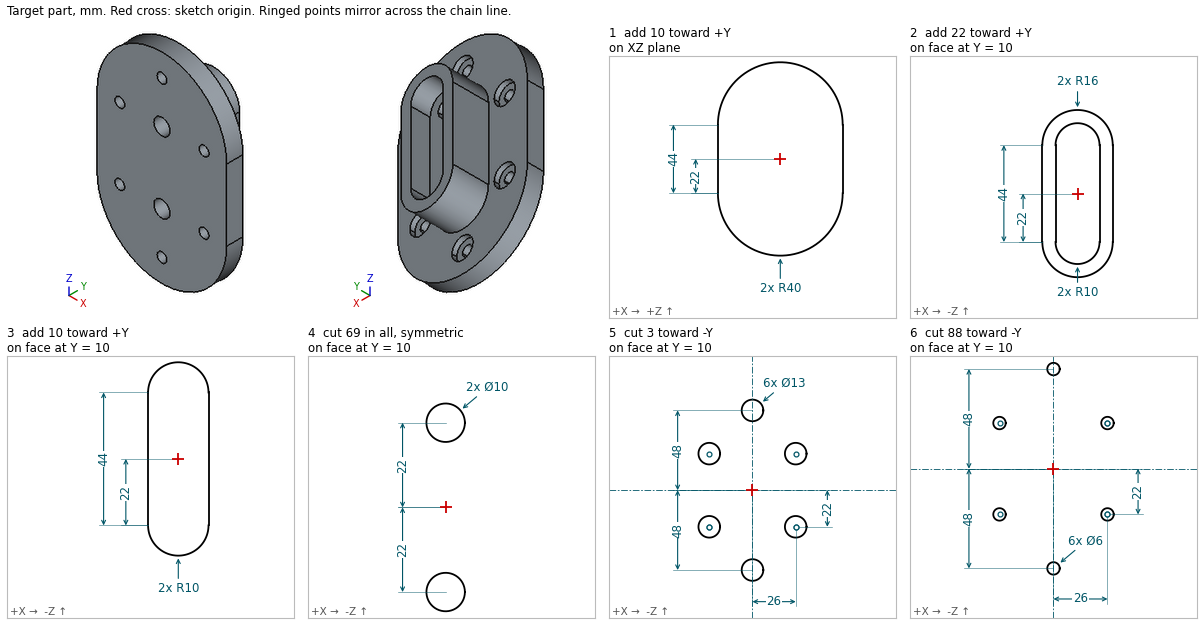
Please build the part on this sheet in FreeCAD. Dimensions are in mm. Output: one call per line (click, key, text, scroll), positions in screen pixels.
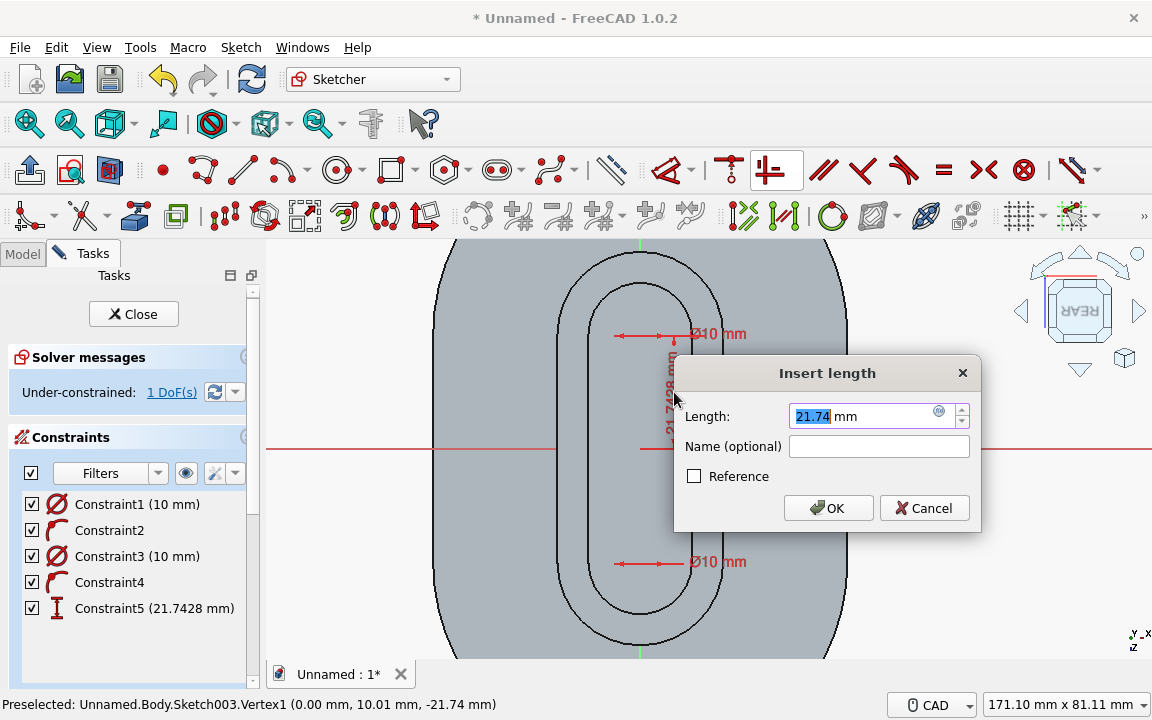
text(22)
key(Return)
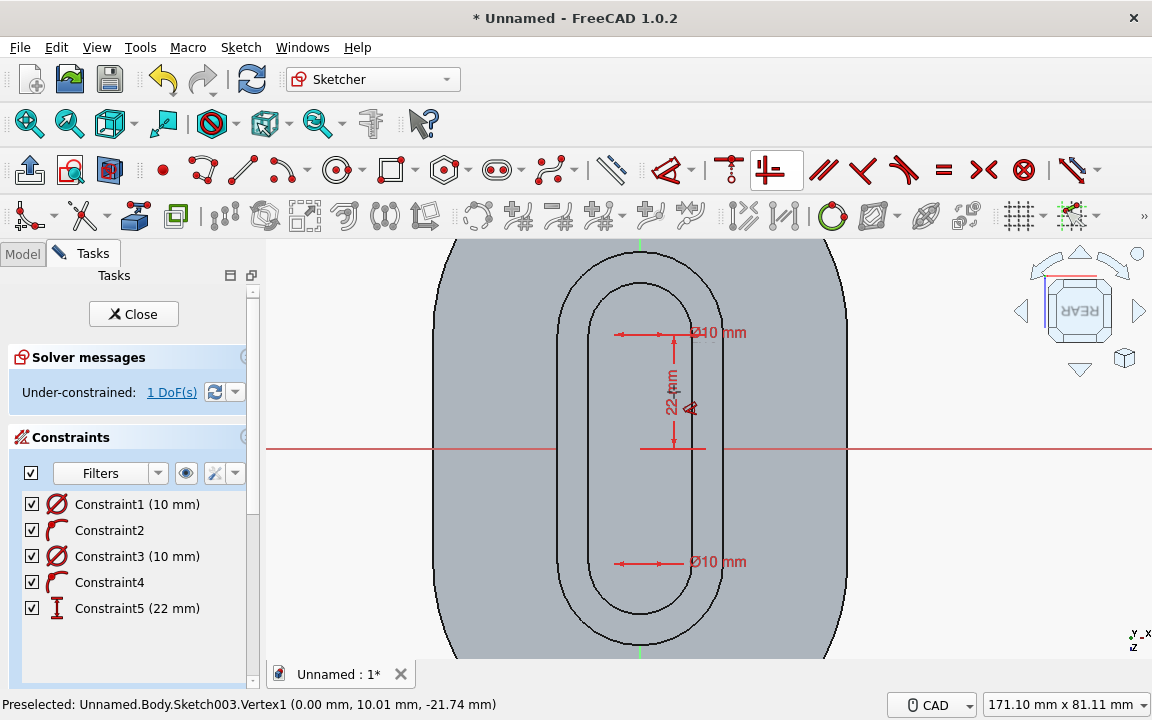
click(640, 564)
click(674, 506)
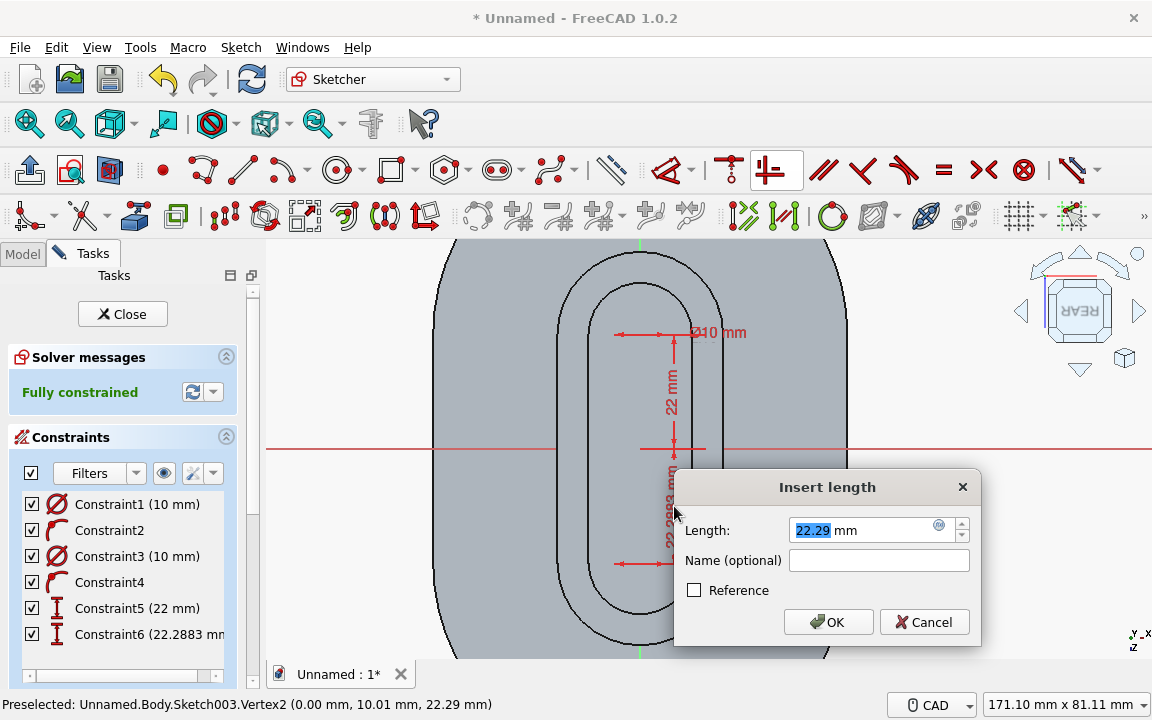
text(22)
key(Return)
key(Escape)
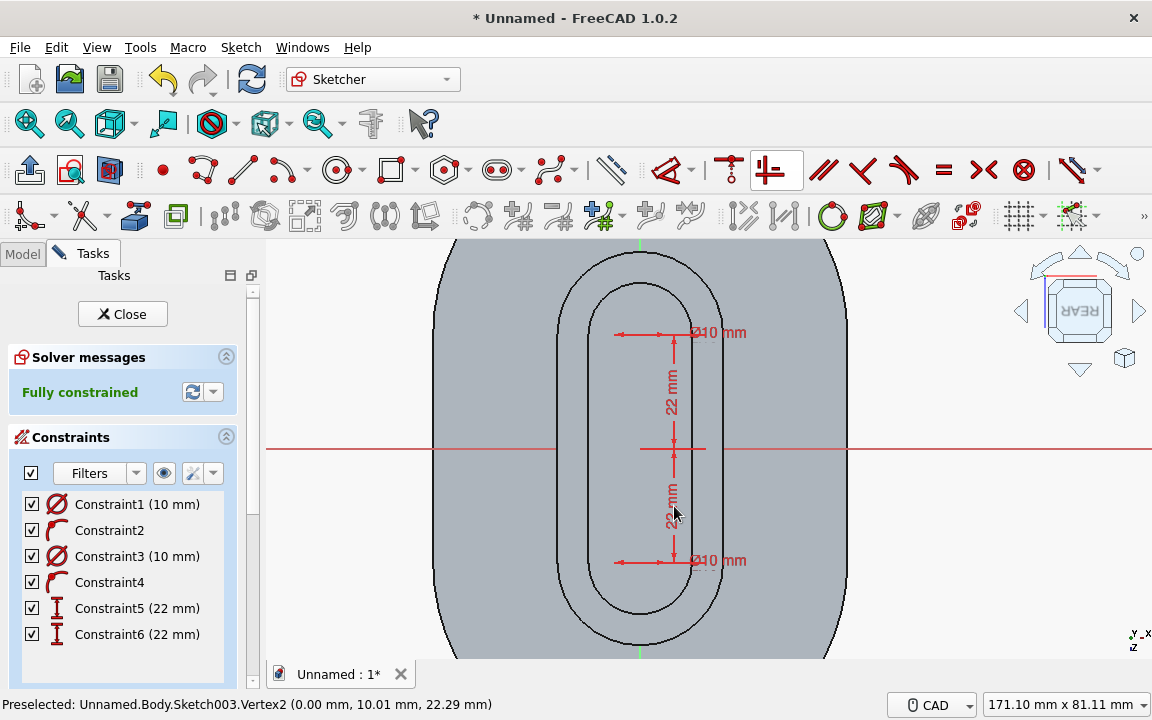
click(123, 314)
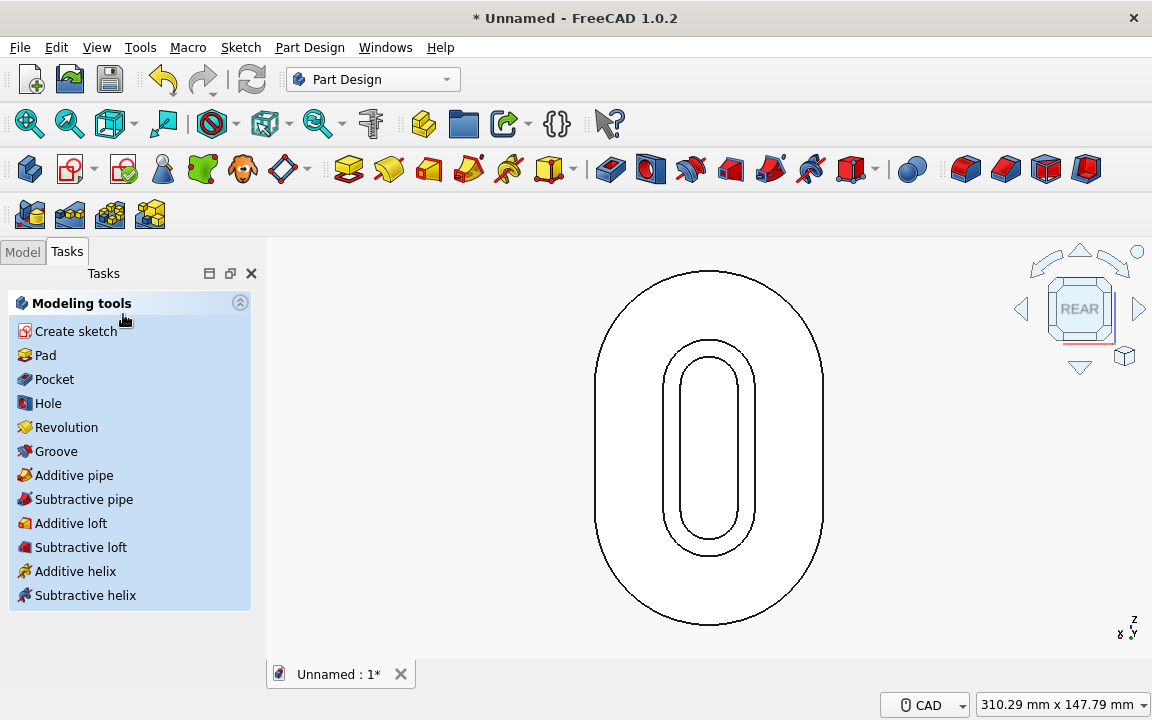
click(612, 170)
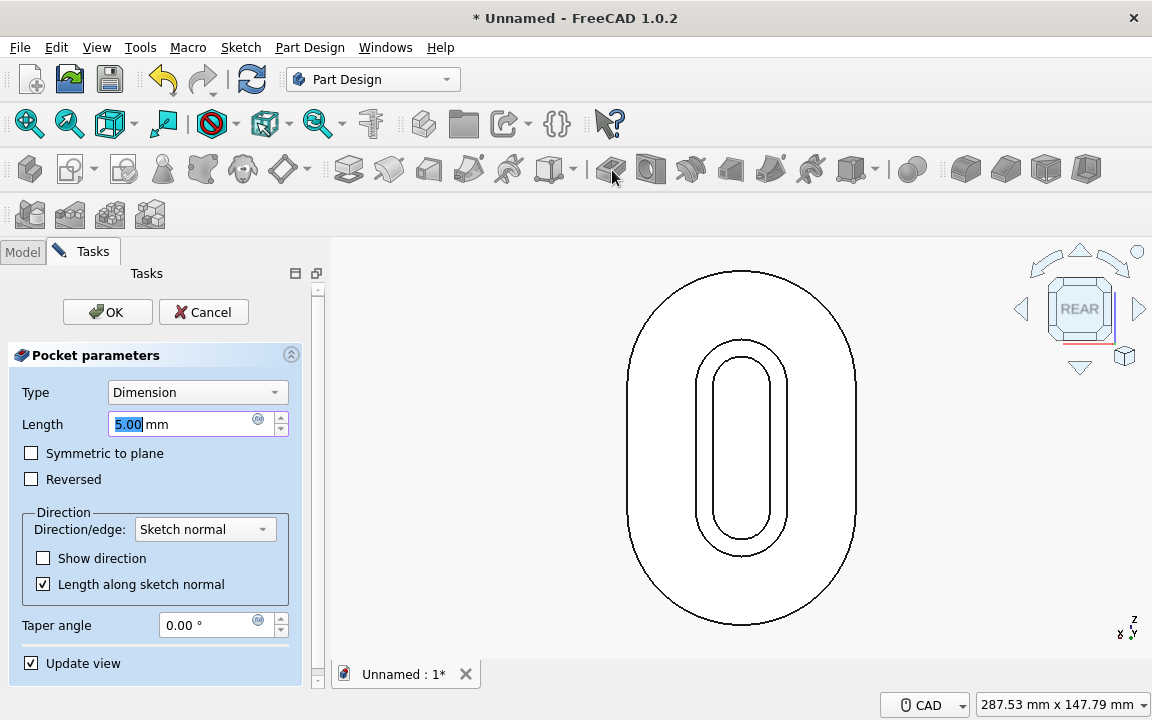
text(69)
key(Tab)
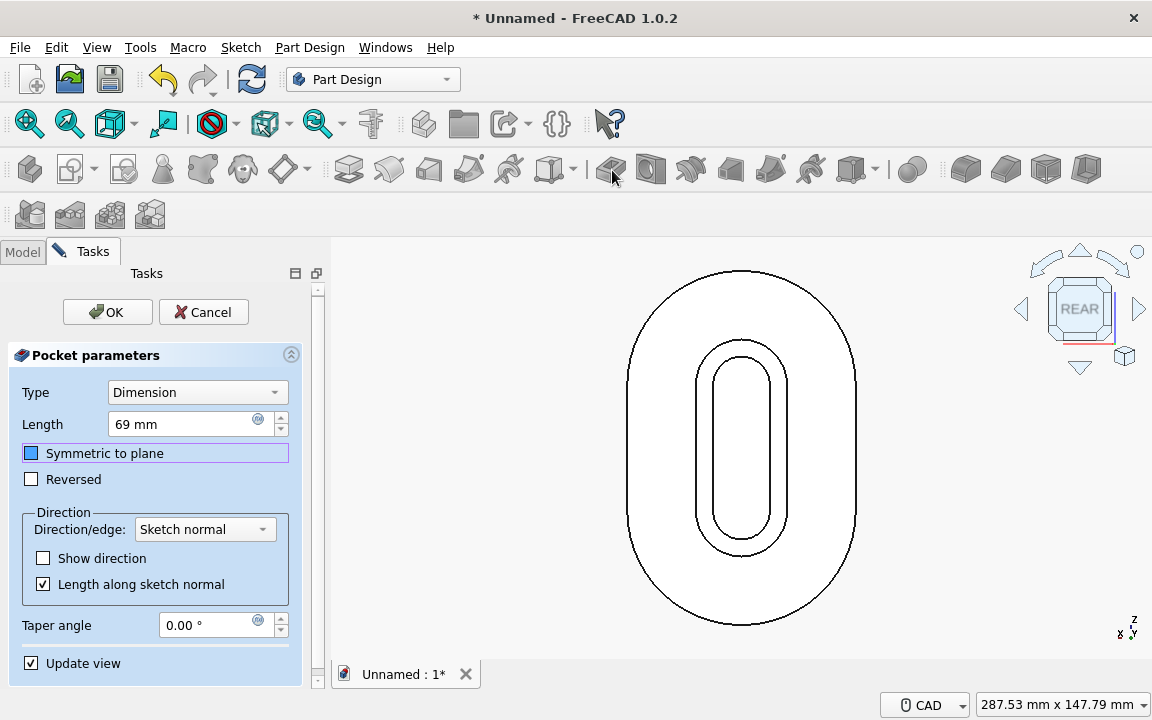
click(30, 453)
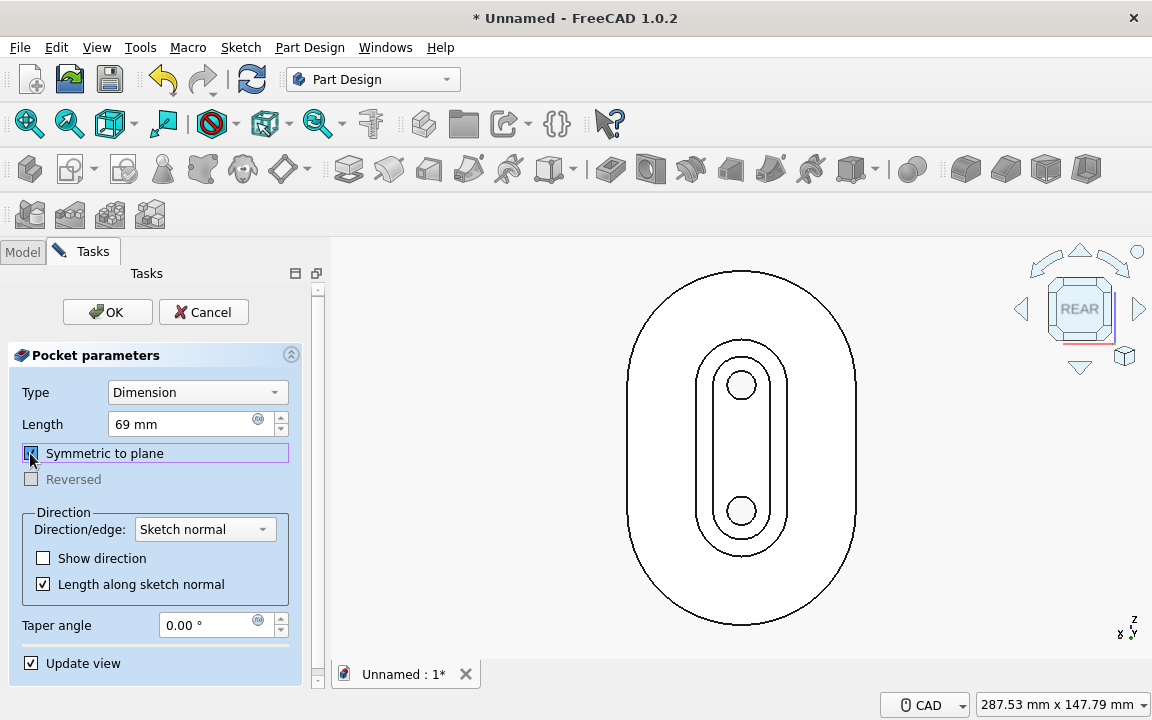
click(108, 312)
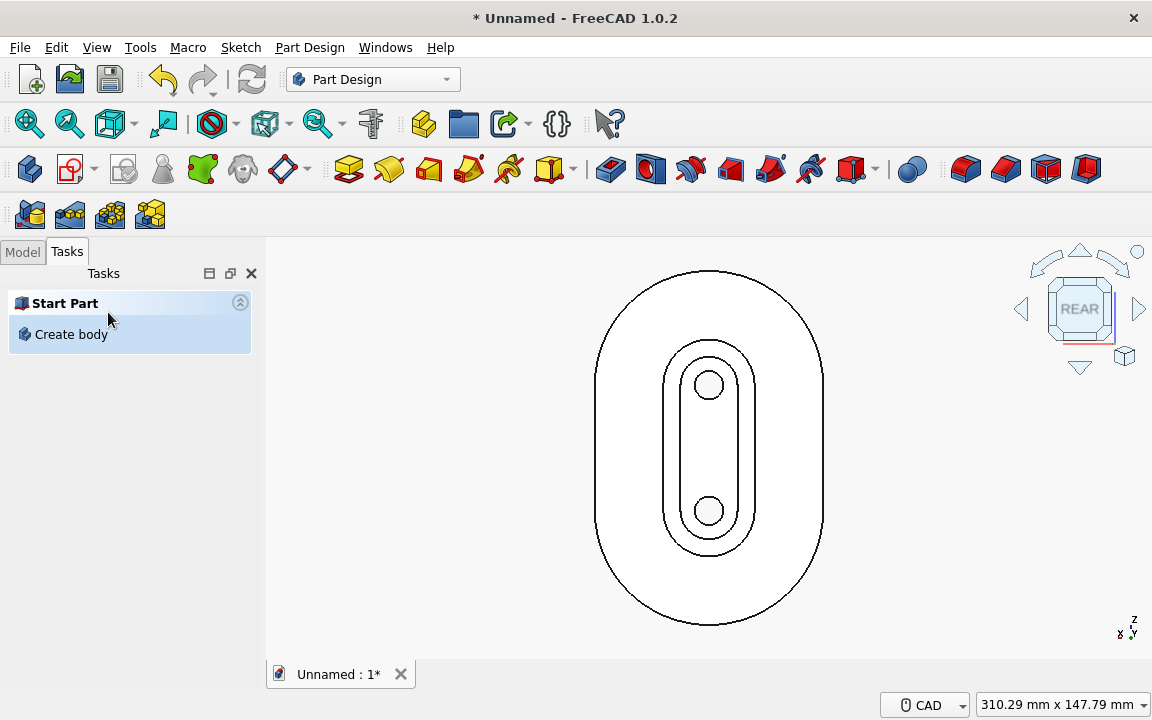
click(644, 548)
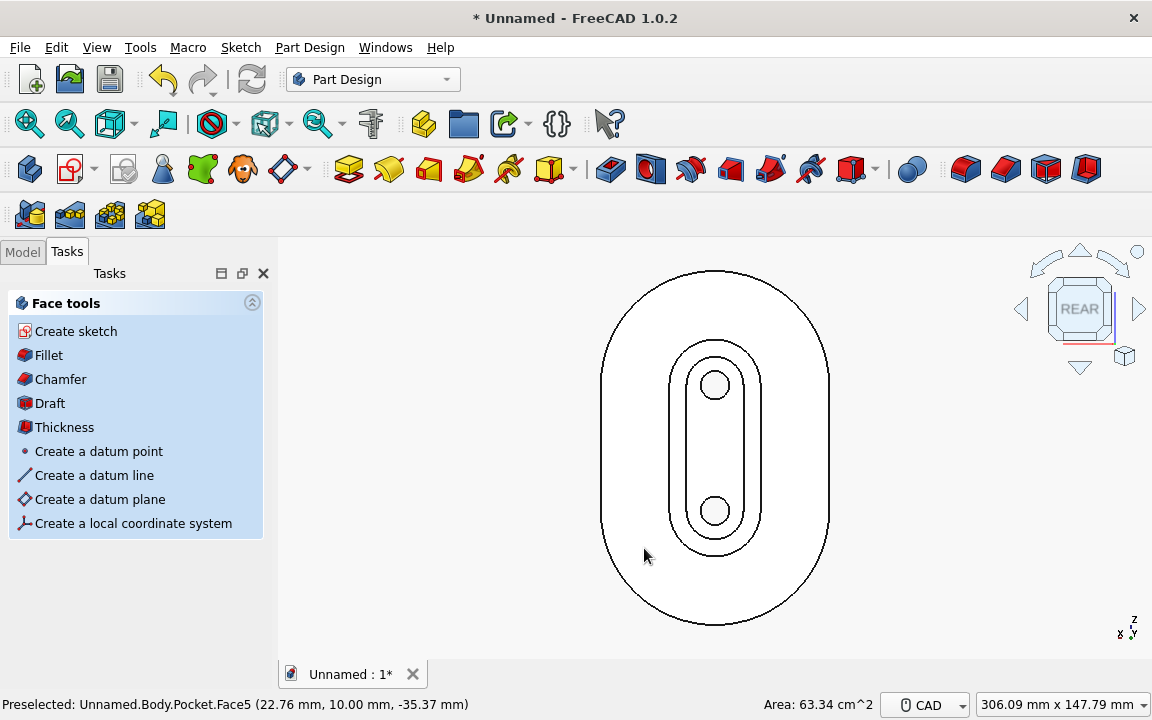
click(70, 170)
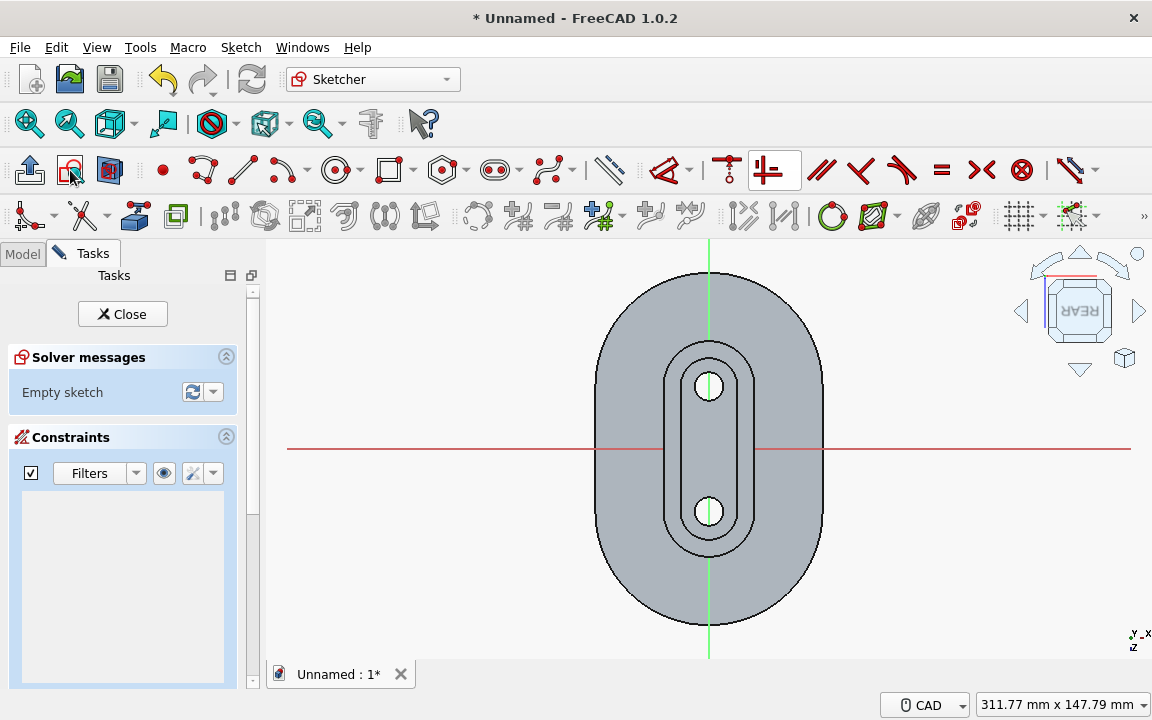
click(336, 170)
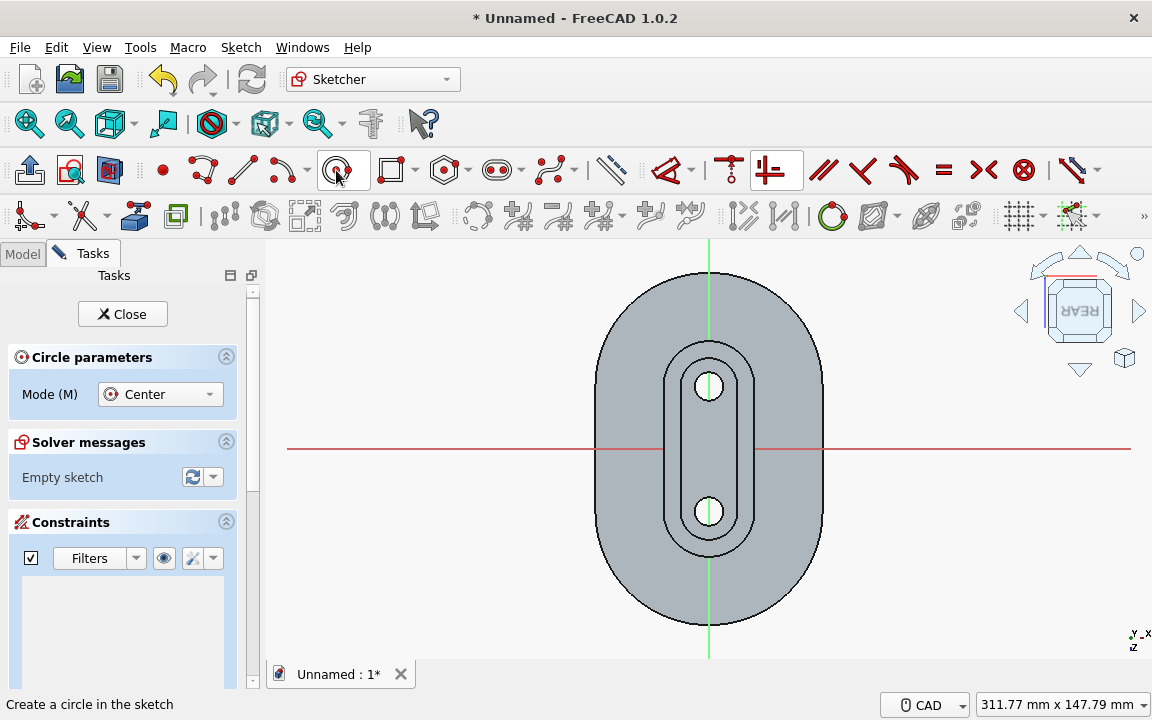
scroll(709, 585, up, 2)